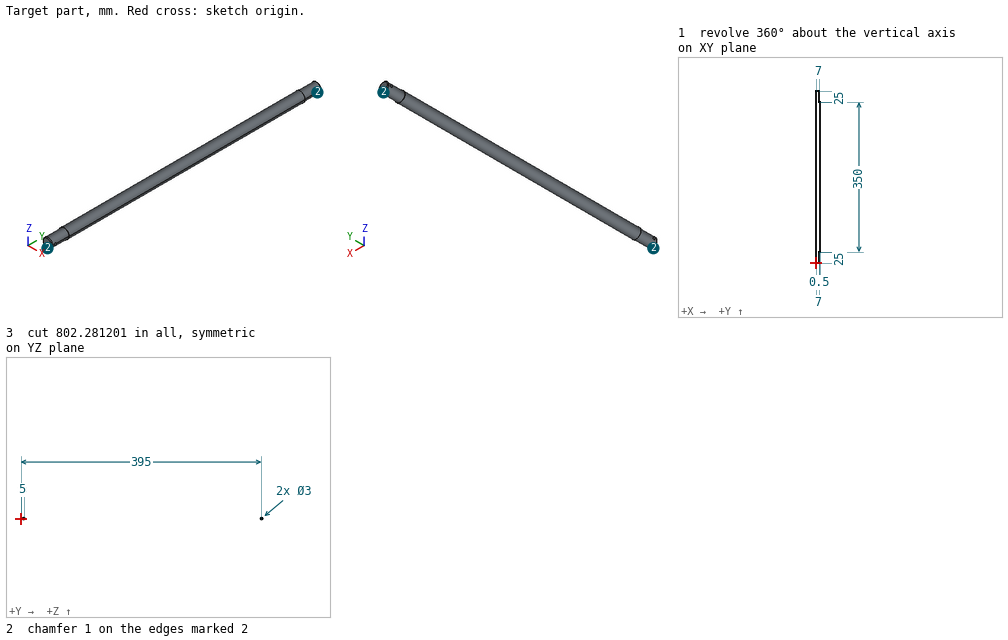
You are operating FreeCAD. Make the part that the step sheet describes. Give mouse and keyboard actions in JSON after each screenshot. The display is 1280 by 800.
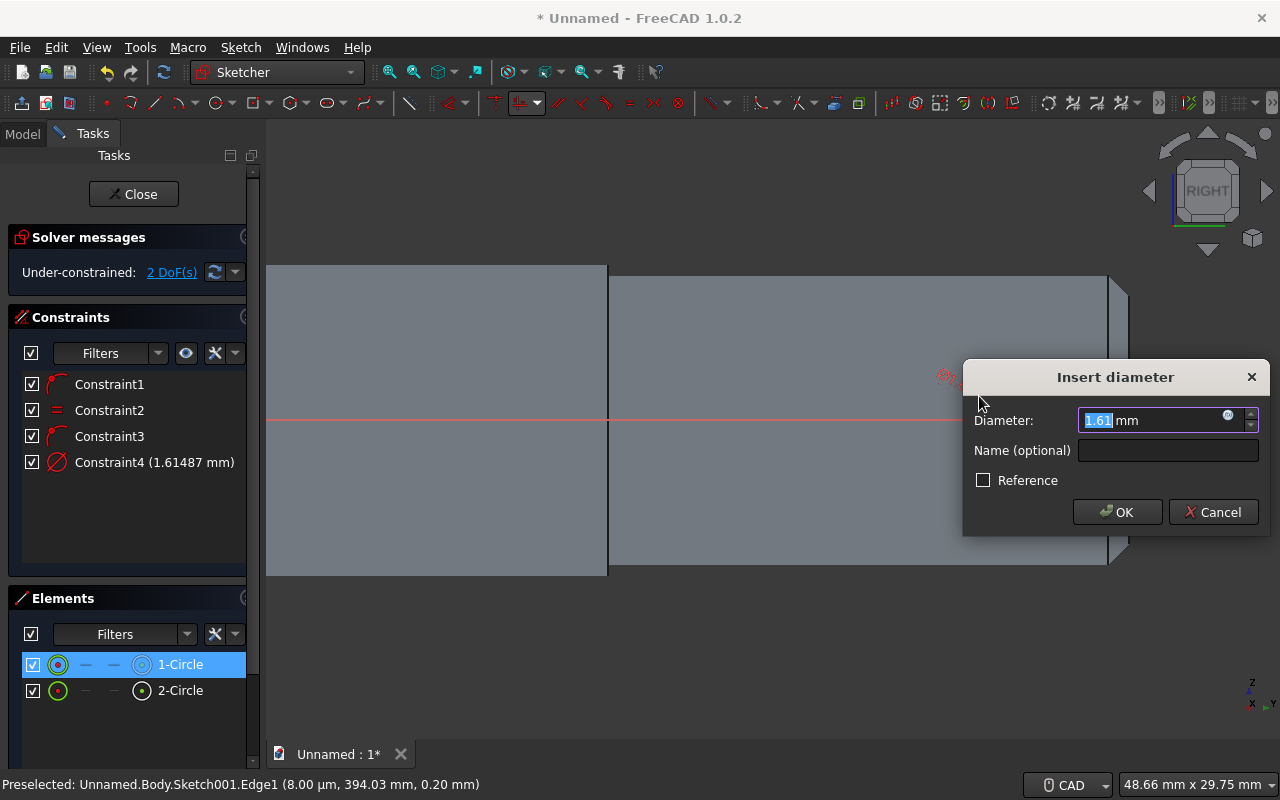
{"action": "type", "text": "3"}
{"action": "key", "text": "Return"}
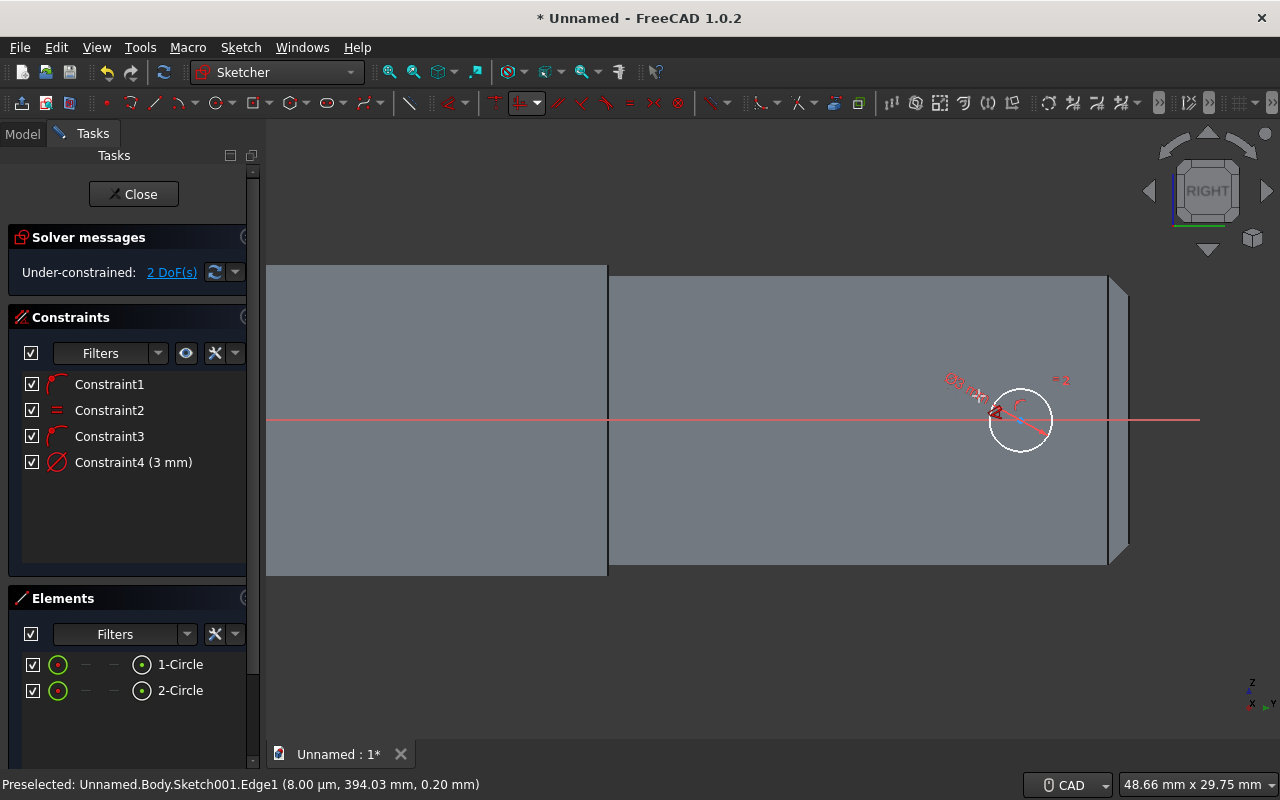
{"action": "scroll", "coordinate": [1008, 430], "scroll_direction": "down", "scroll_amount": 13}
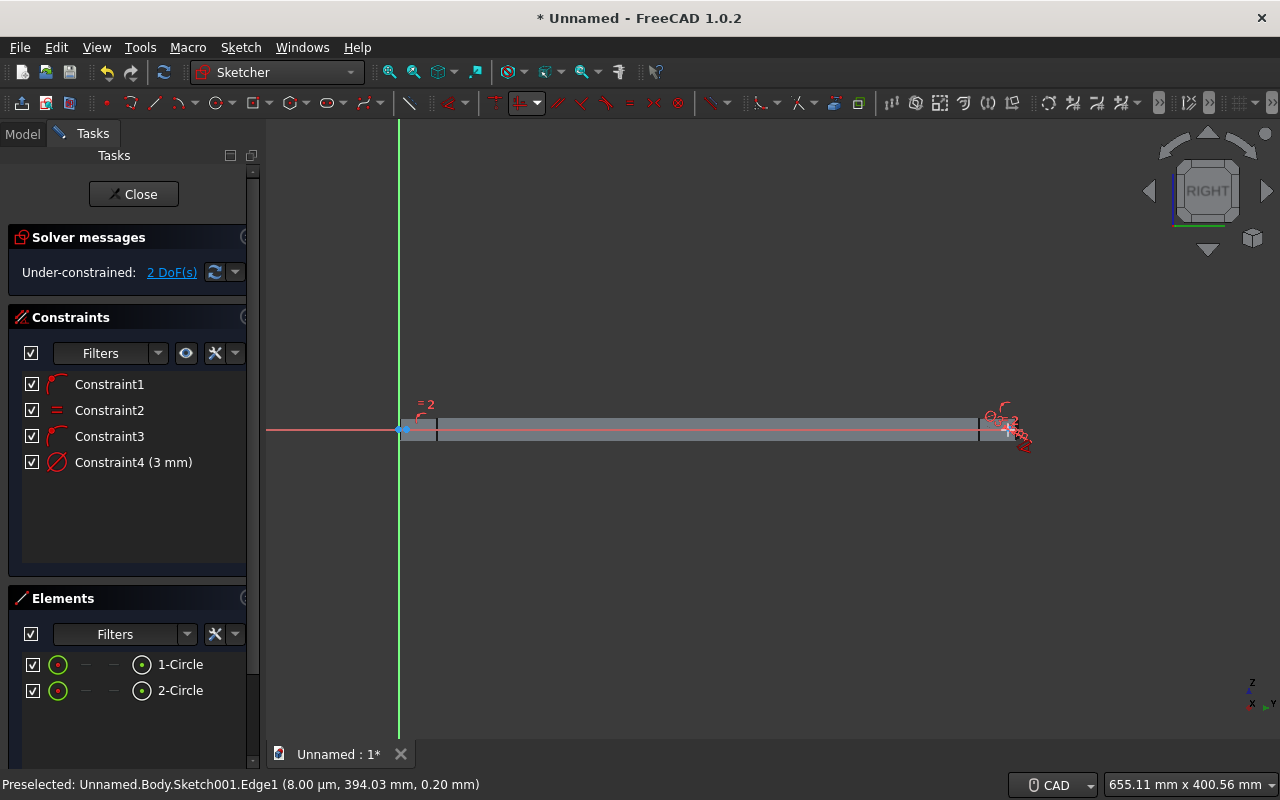
{"action": "scroll", "coordinate": [406, 430], "scroll_direction": "up", "scroll_amount": 9}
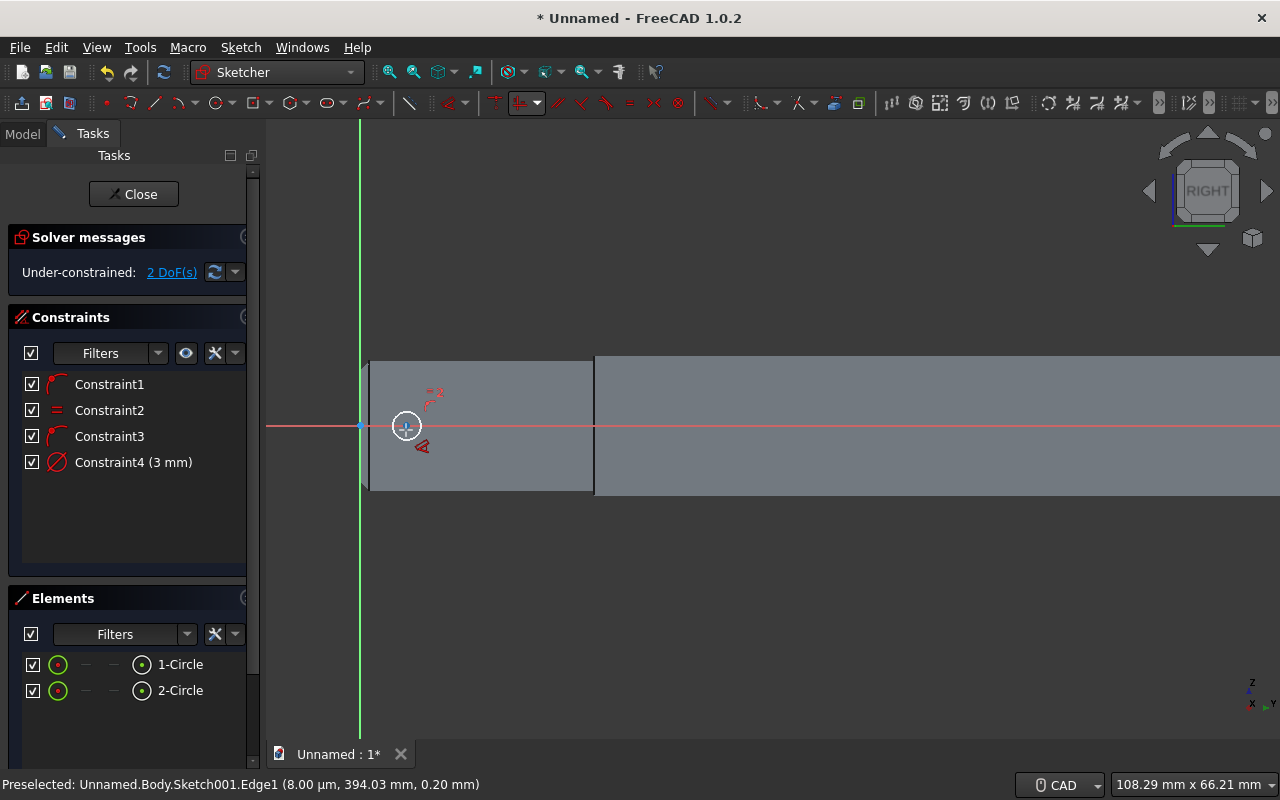
{"action": "left_click", "coordinate": [407, 426]}
{"action": "left_click", "coordinate": [383, 460]}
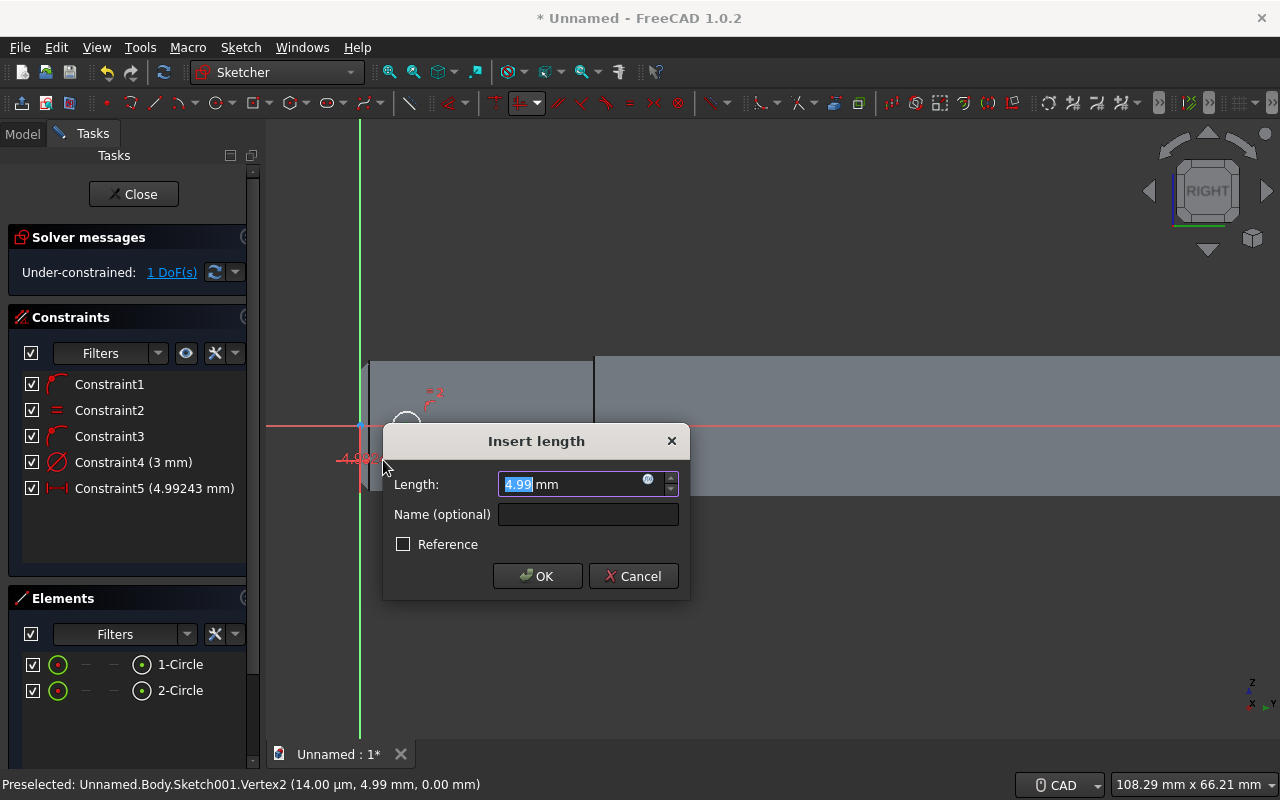
{"action": "type", "text": "5"}
{"action": "key", "text": "Return"}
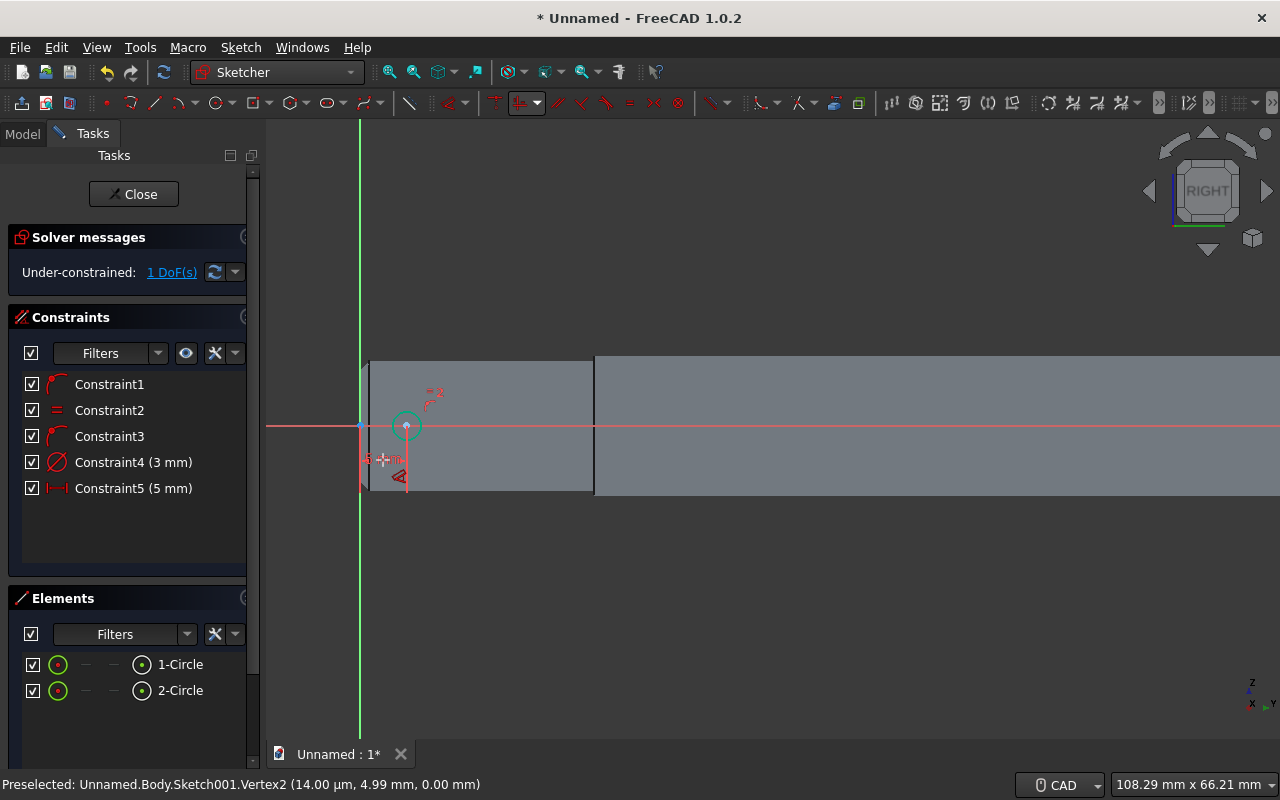
{"action": "scroll", "coordinate": [405, 430], "scroll_direction": "down", "scroll_amount": 9}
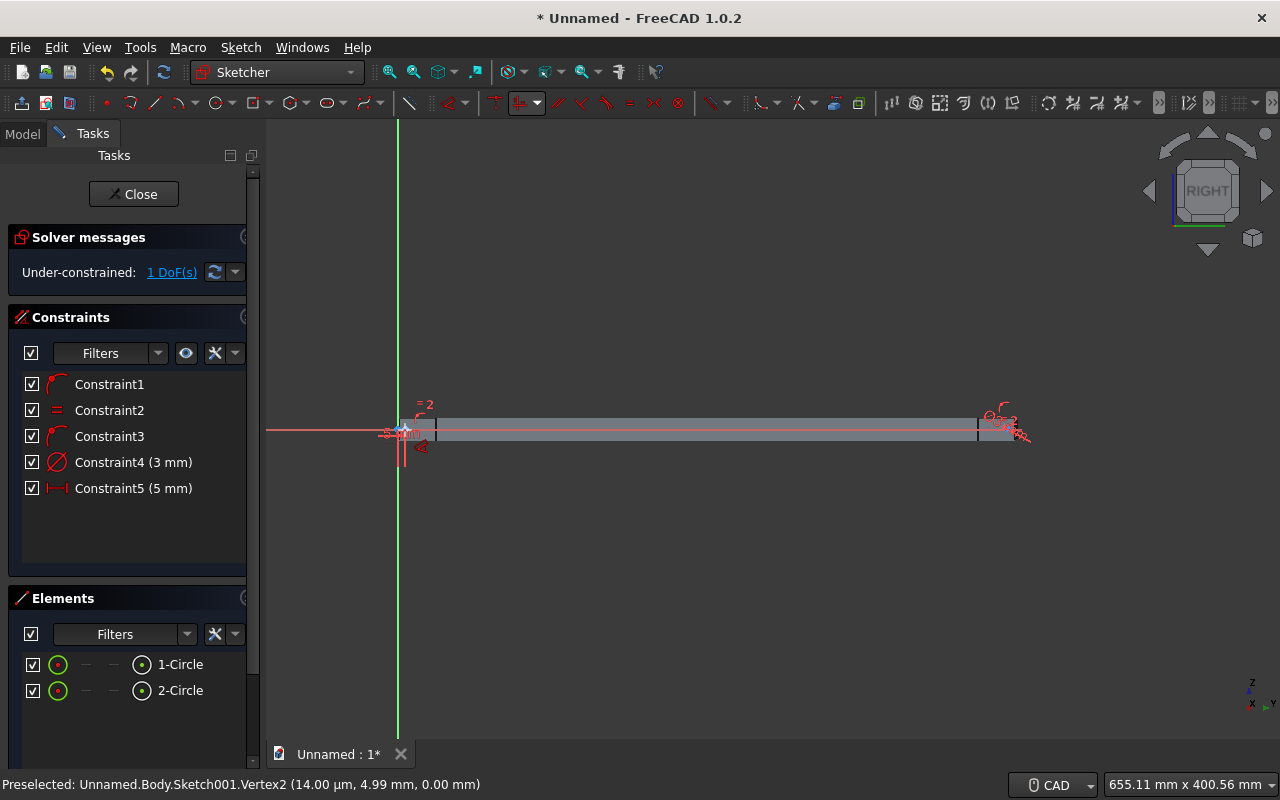
{"action": "left_click", "coordinate": [1009, 430]}
{"action": "left_click", "coordinate": [703, 464]}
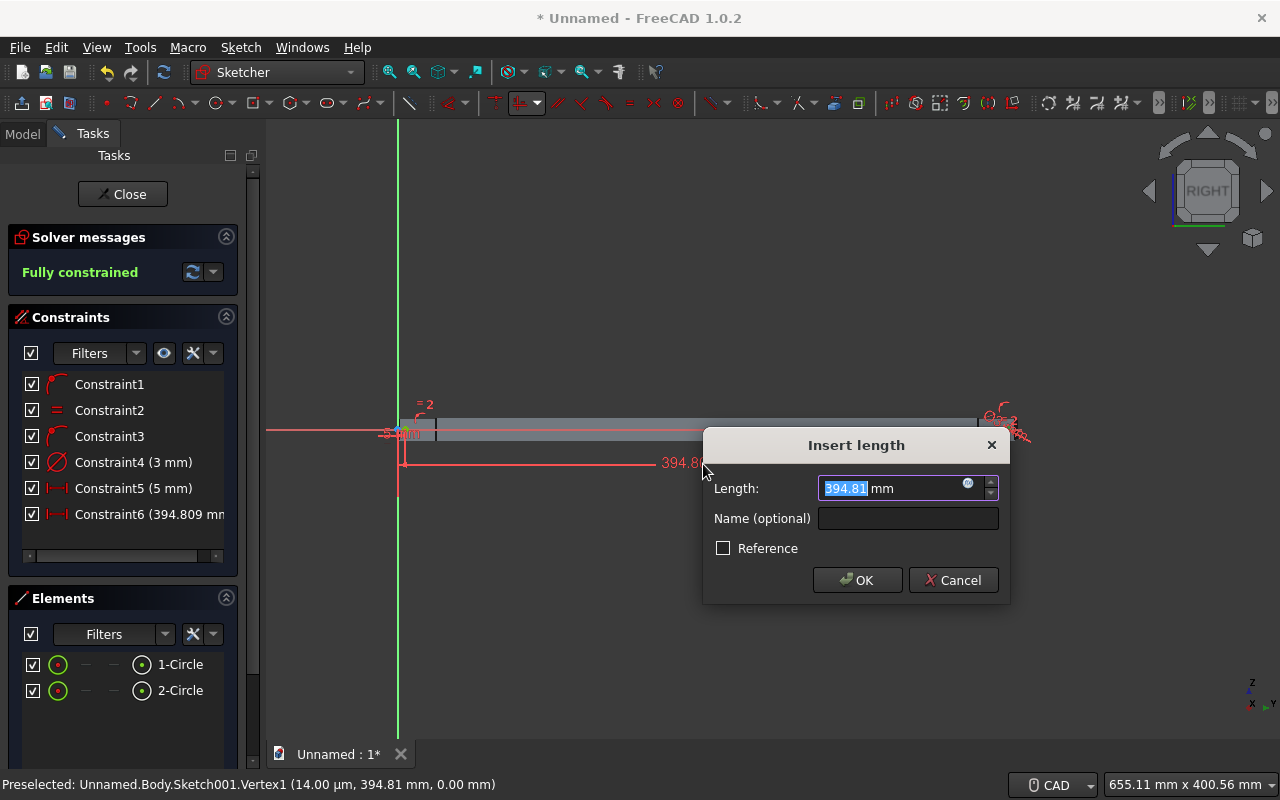
{"action": "type", "text": "395"}
{"action": "key", "text": "Return"}
{"action": "key", "text": "Escape"}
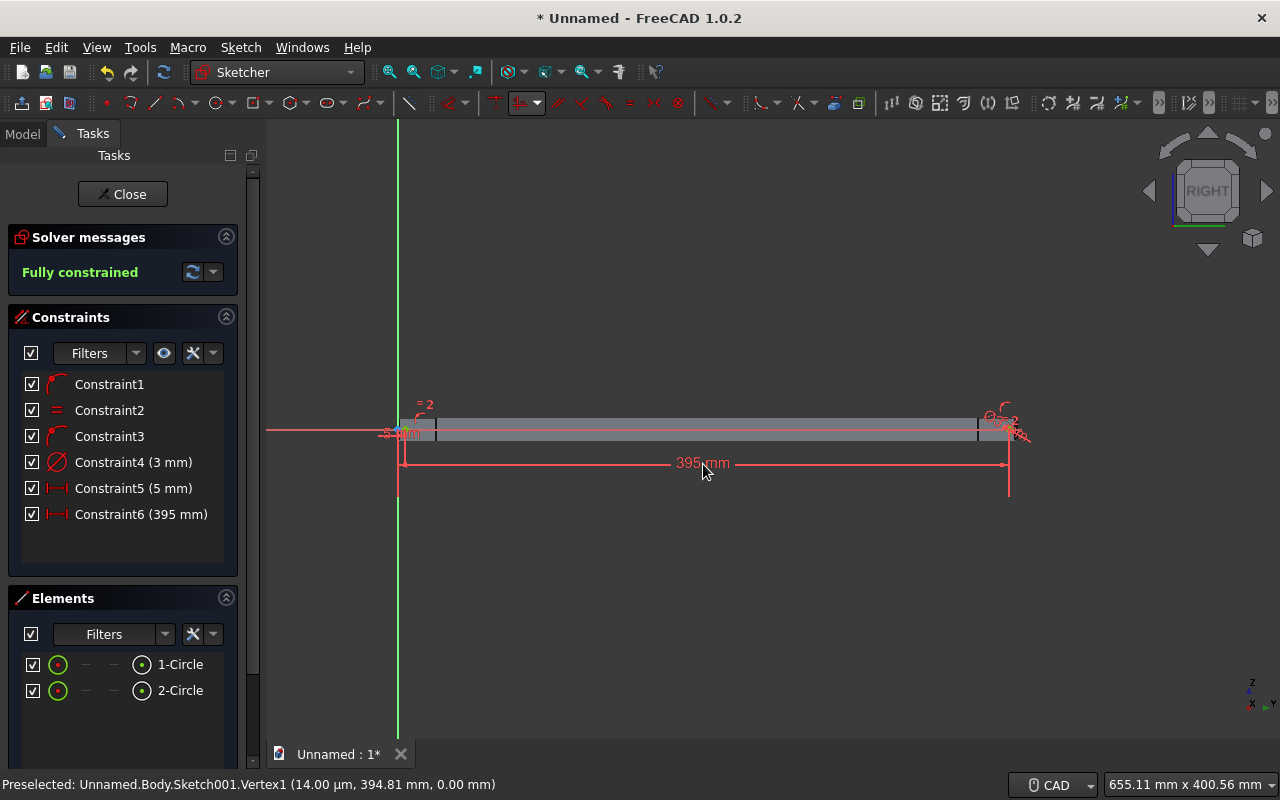
{"action": "left_click", "coordinate": [123, 194]}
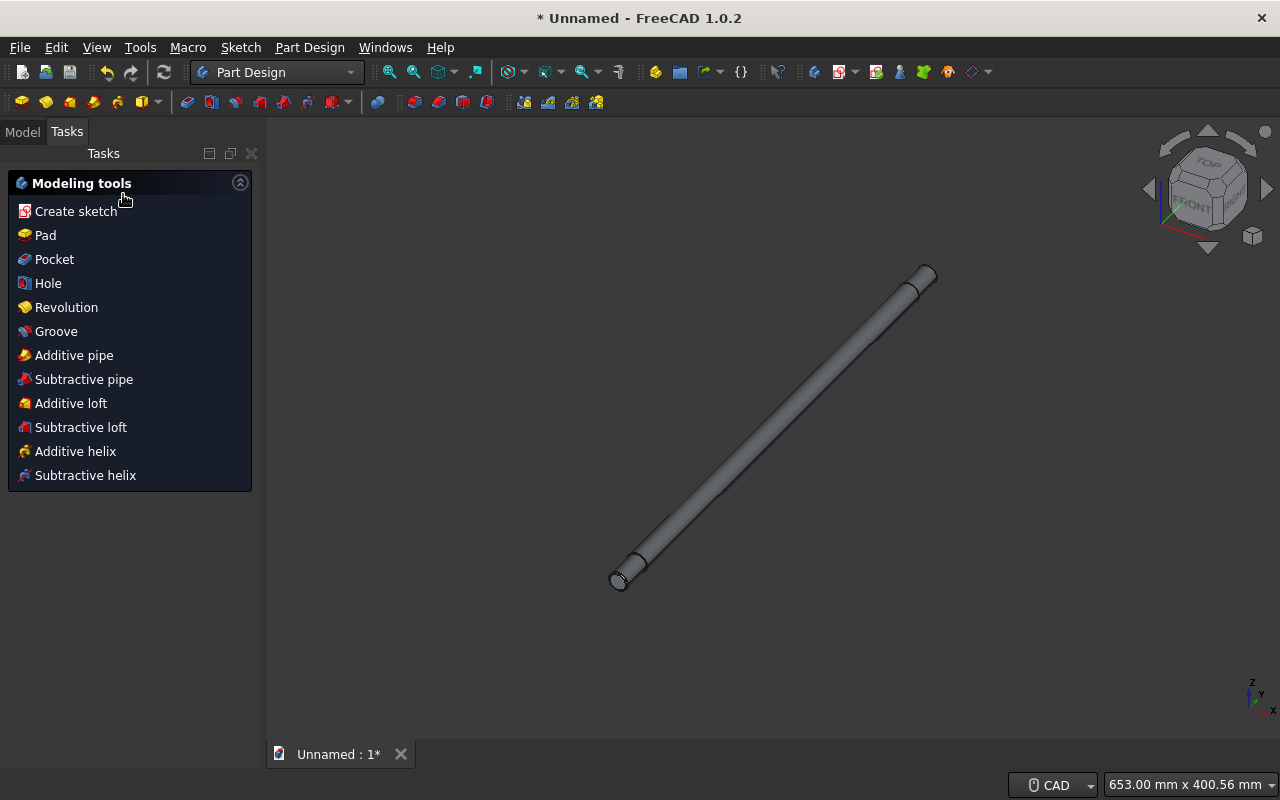
{"action": "left_click", "coordinate": [188, 102]}